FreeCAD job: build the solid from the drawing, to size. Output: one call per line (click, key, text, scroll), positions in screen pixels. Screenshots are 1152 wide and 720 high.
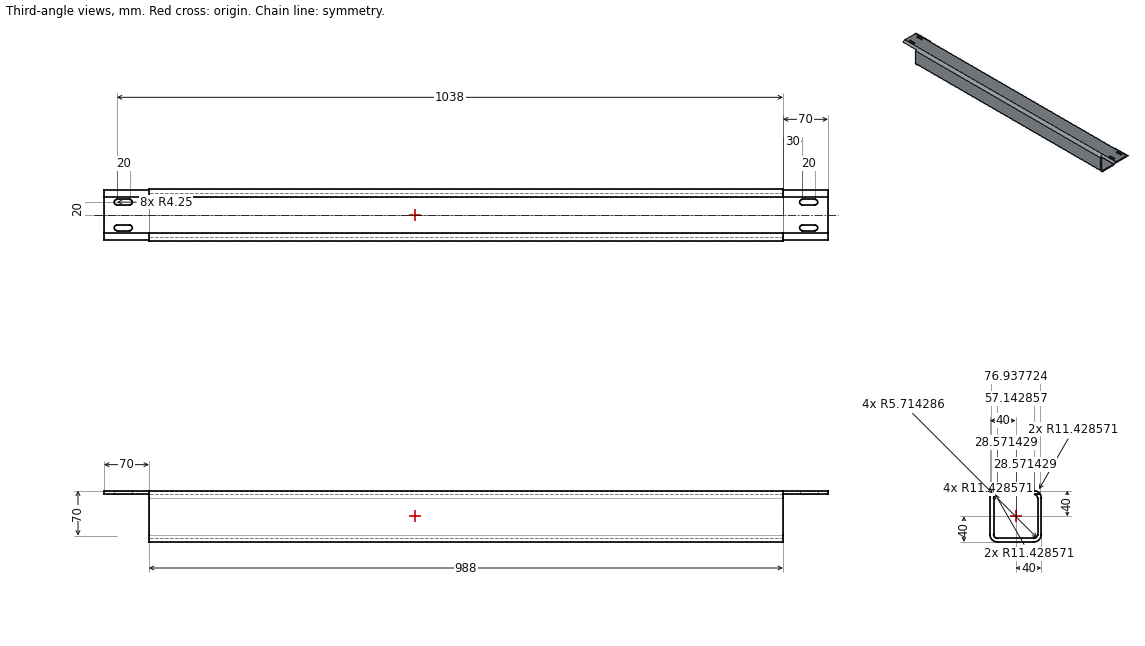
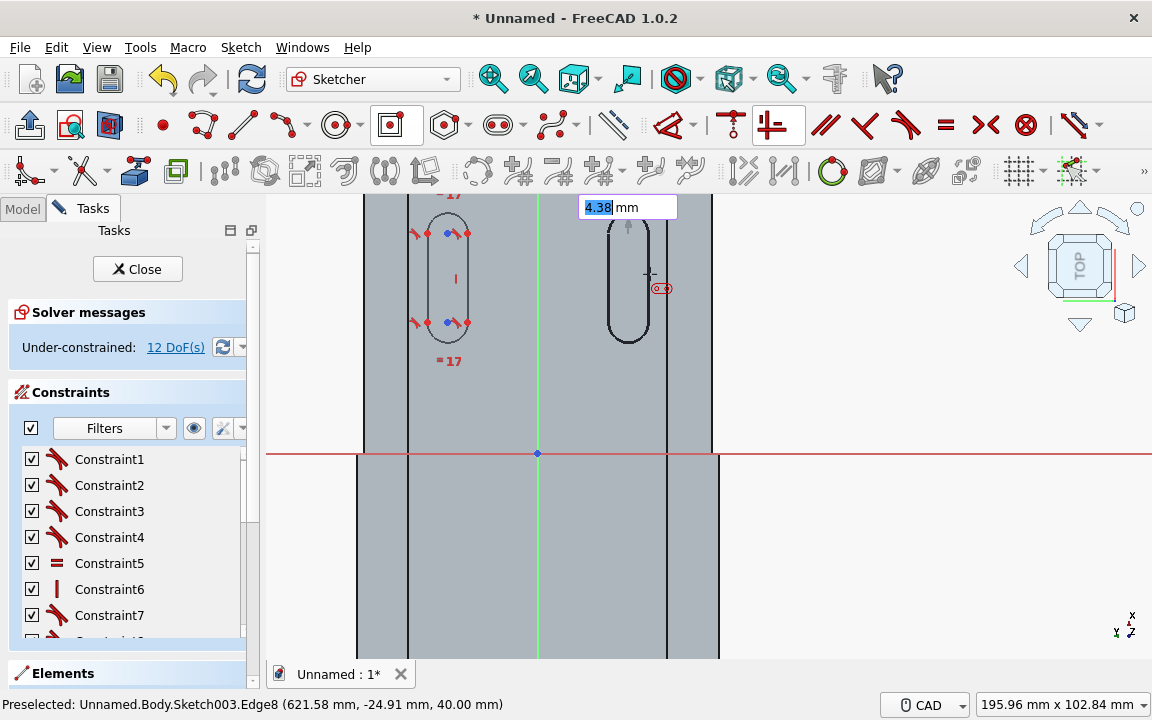
click(647, 273)
key(Escape)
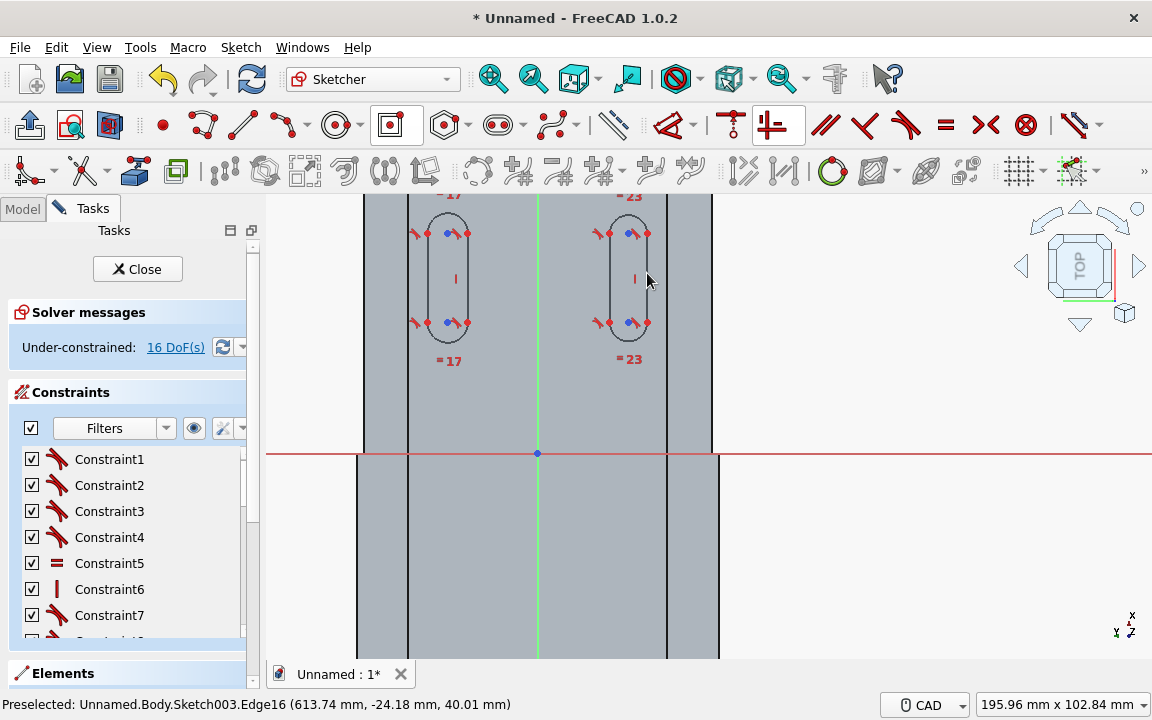
scroll(647, 280, down, 14)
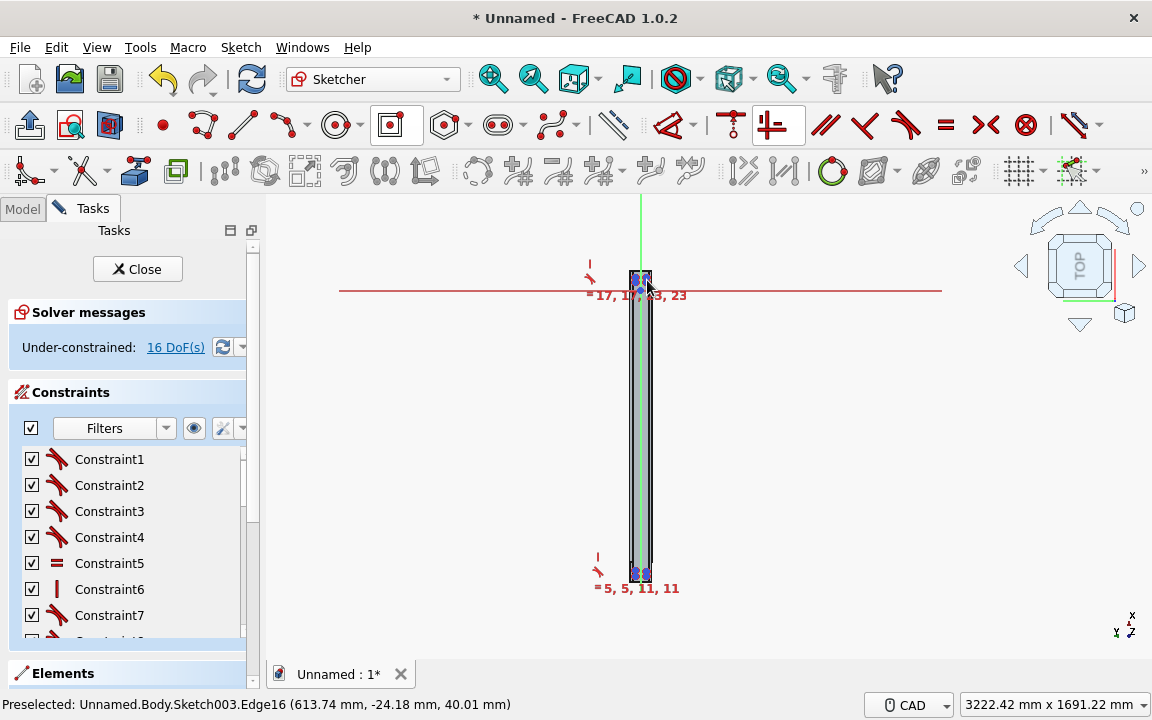
scroll(635, 577, up, 13)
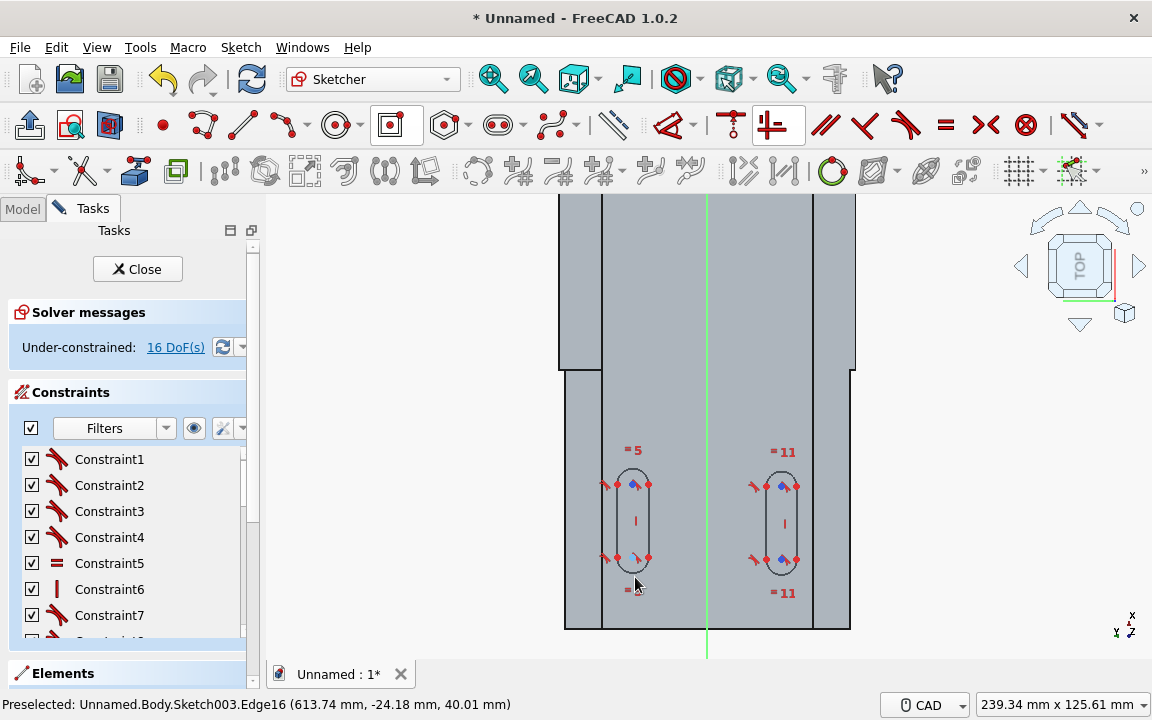
click(624, 570)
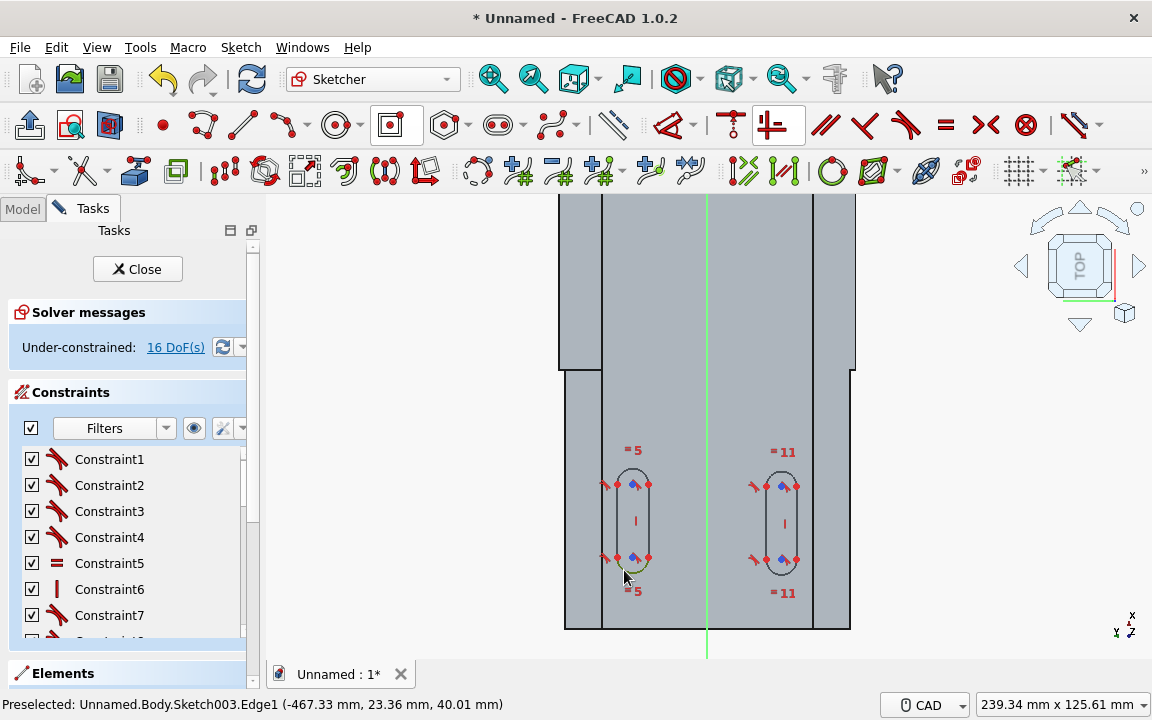
click(773, 572)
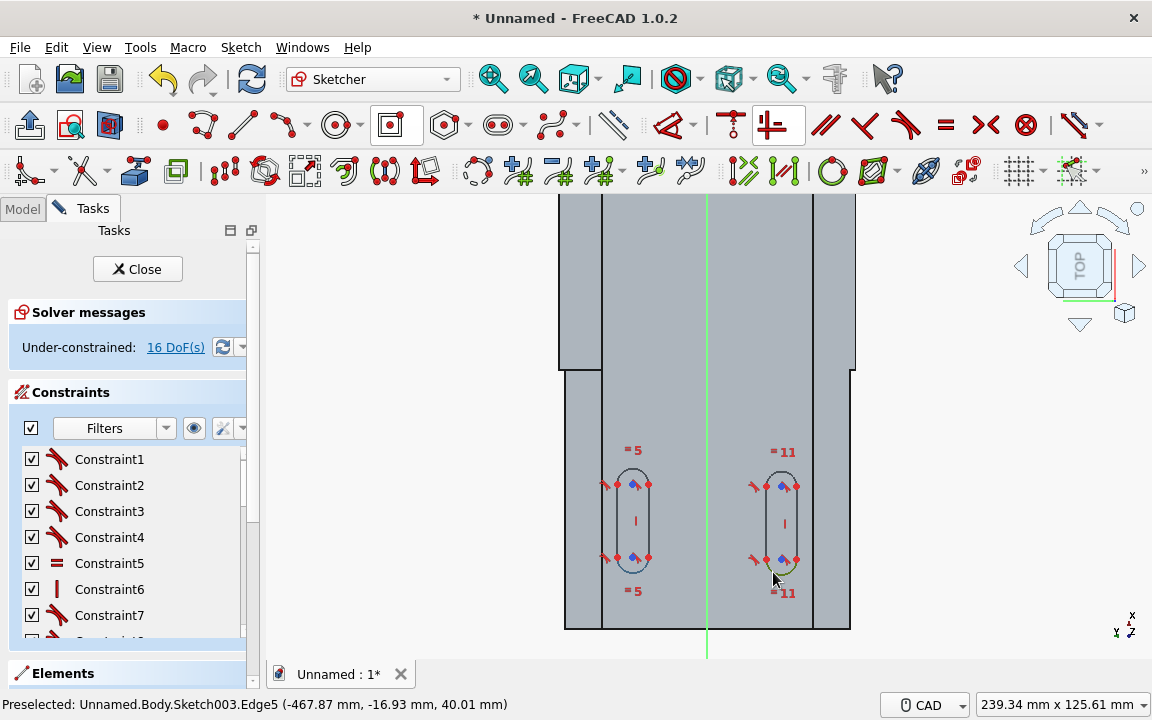
scroll(635, 578, down, 13)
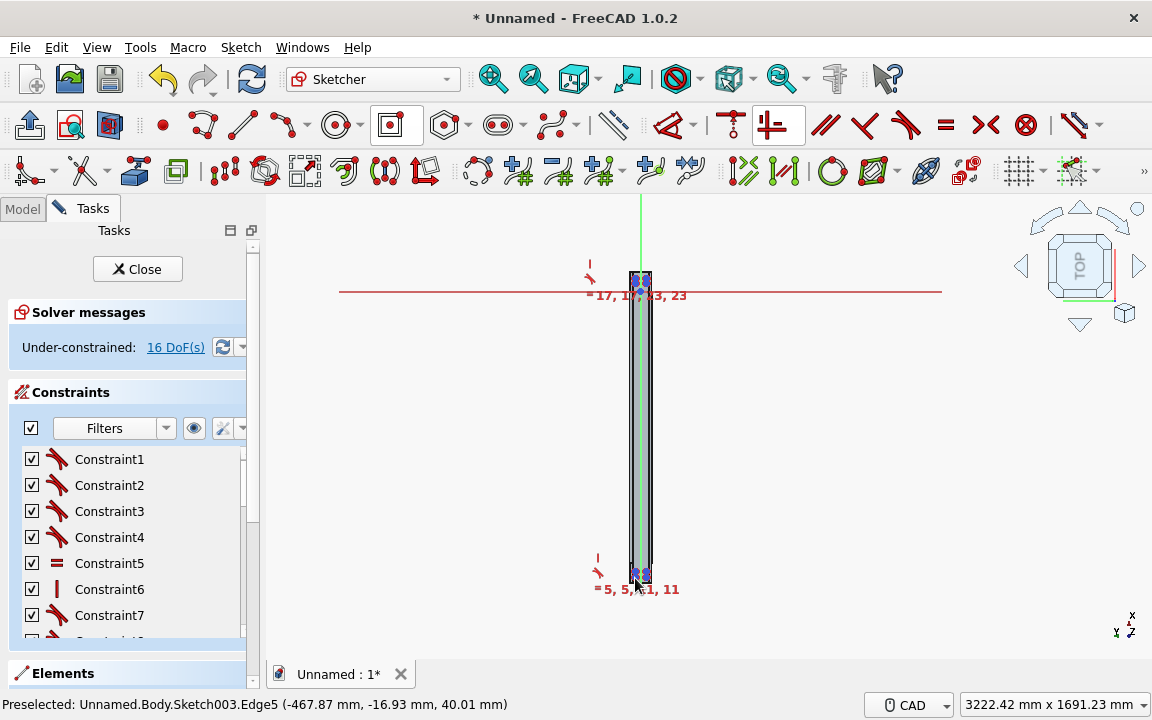
scroll(635, 285, up, 13)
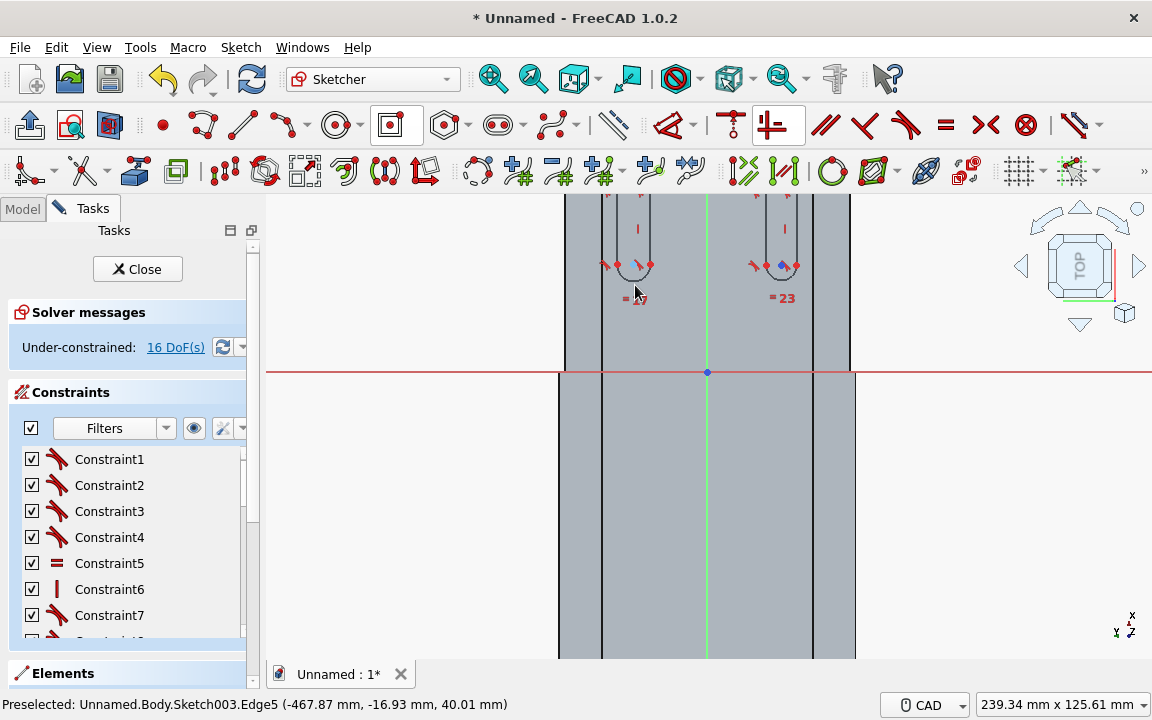
click(624, 278)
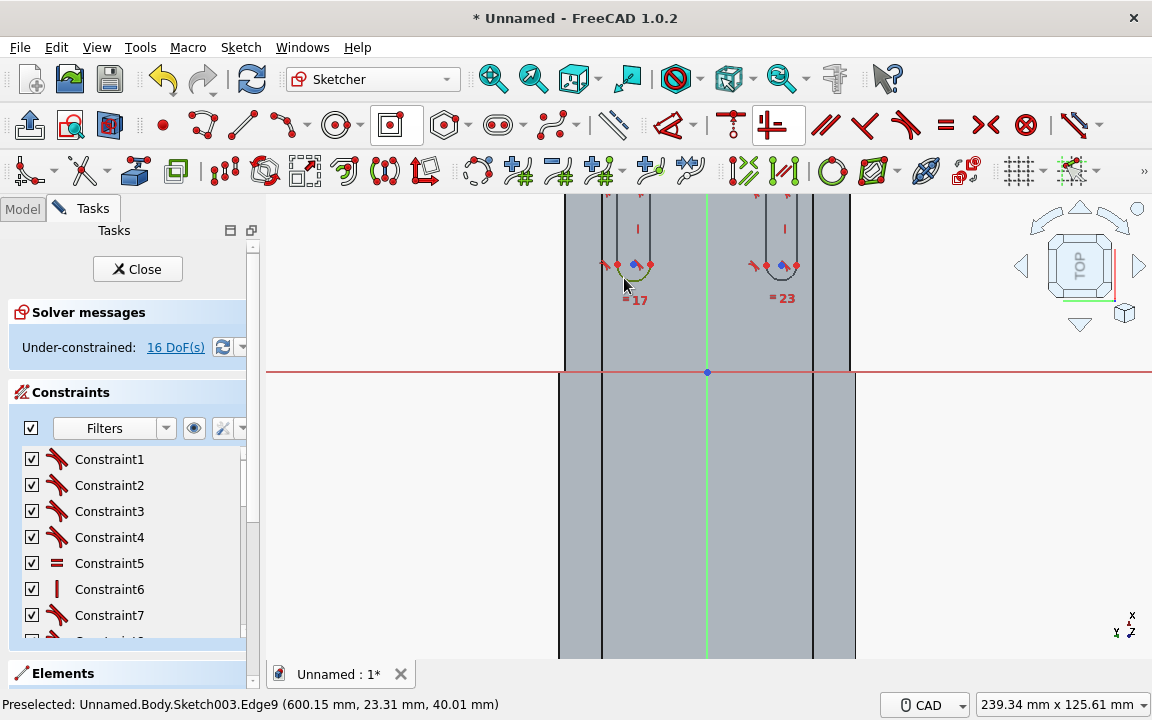
click(773, 277)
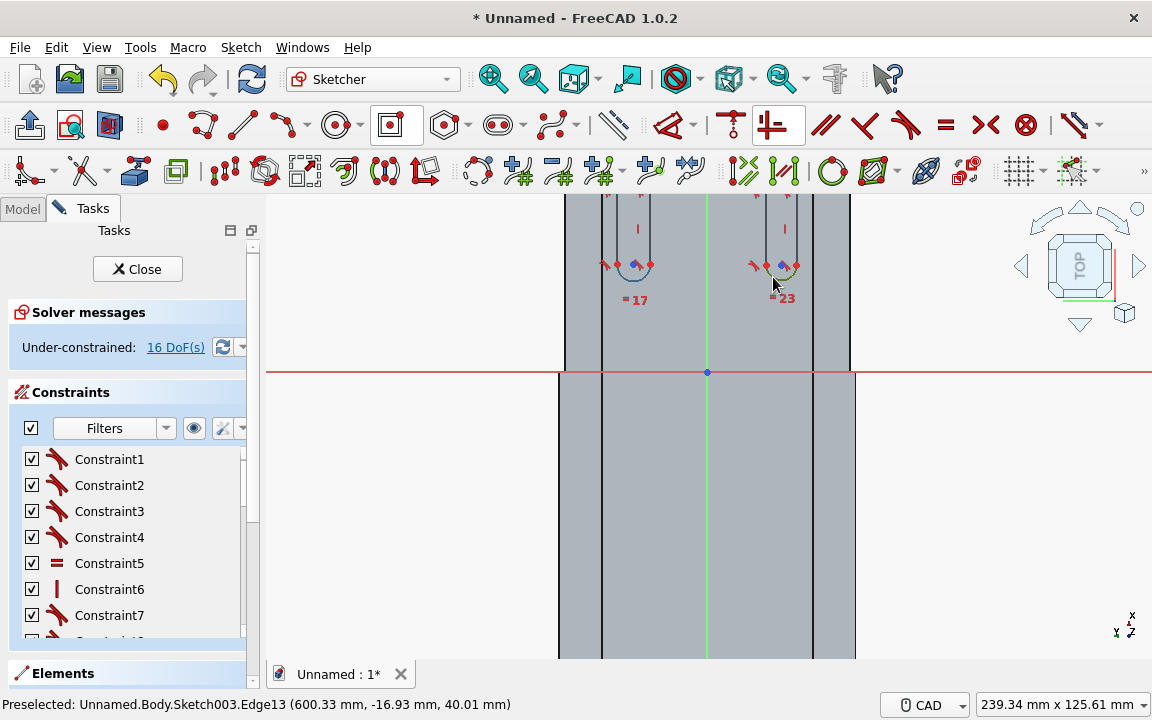
key(e)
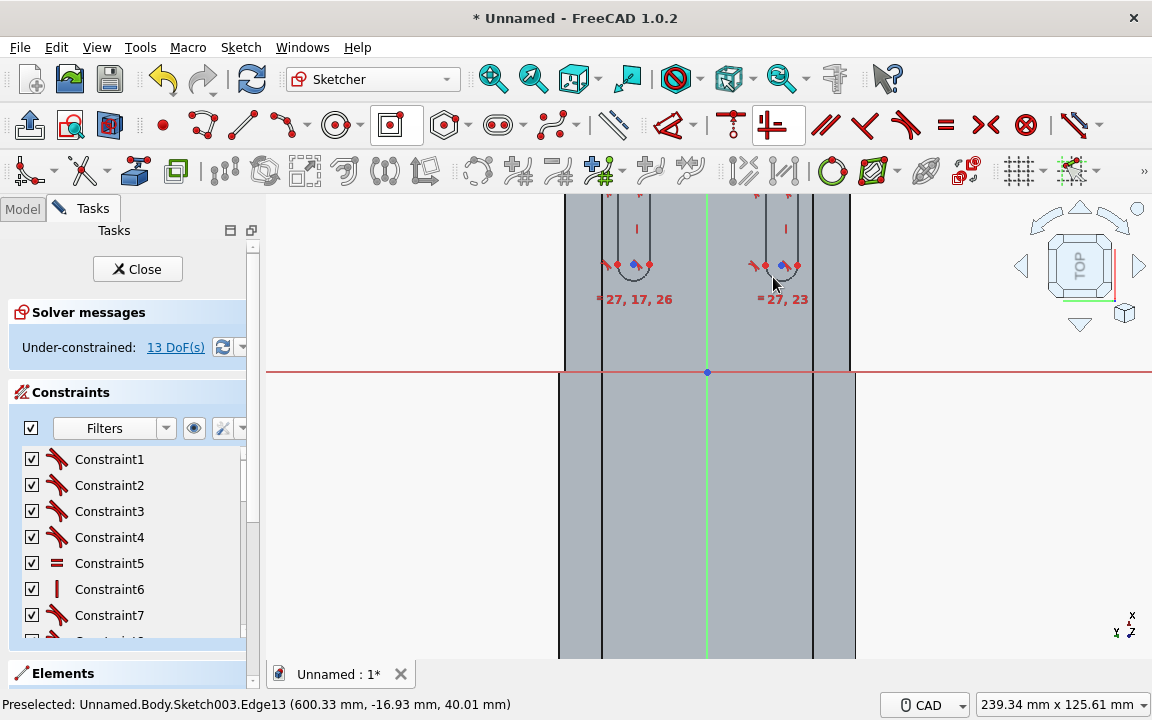
scroll(635, 284, down, 13)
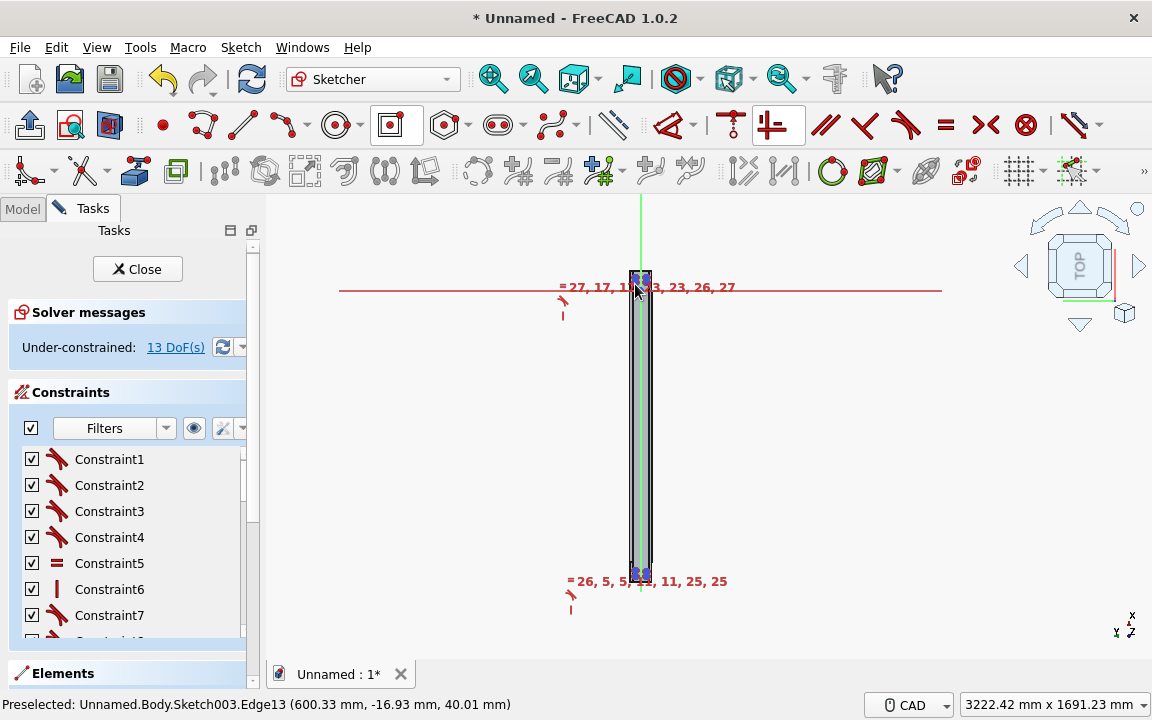
scroll(635, 576, up, 12)